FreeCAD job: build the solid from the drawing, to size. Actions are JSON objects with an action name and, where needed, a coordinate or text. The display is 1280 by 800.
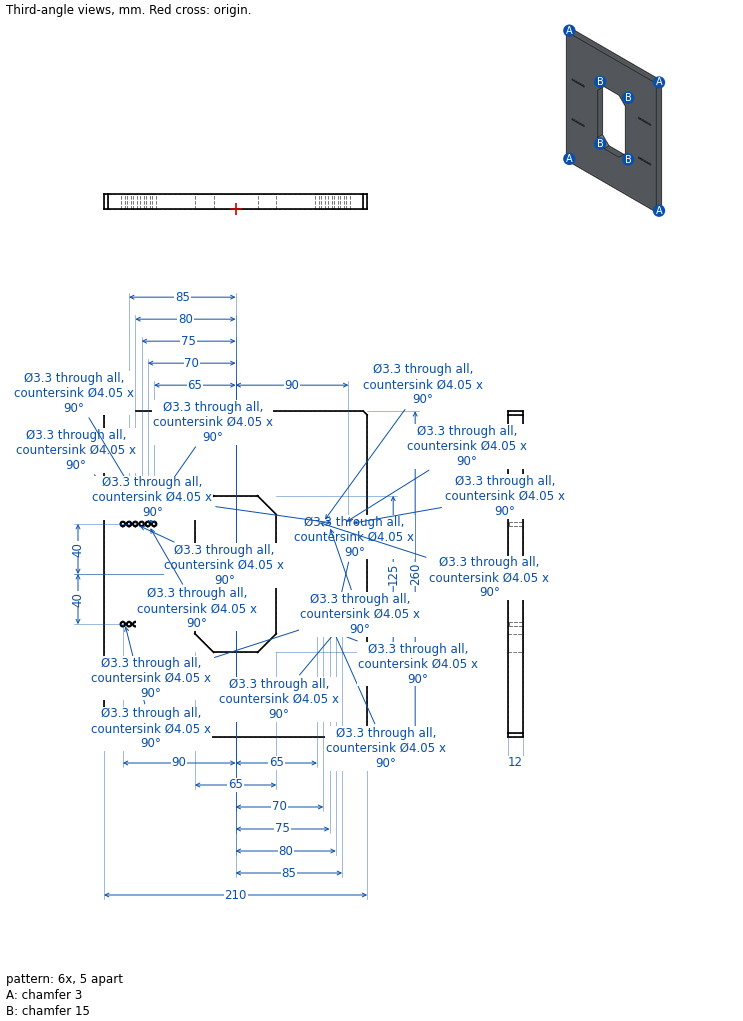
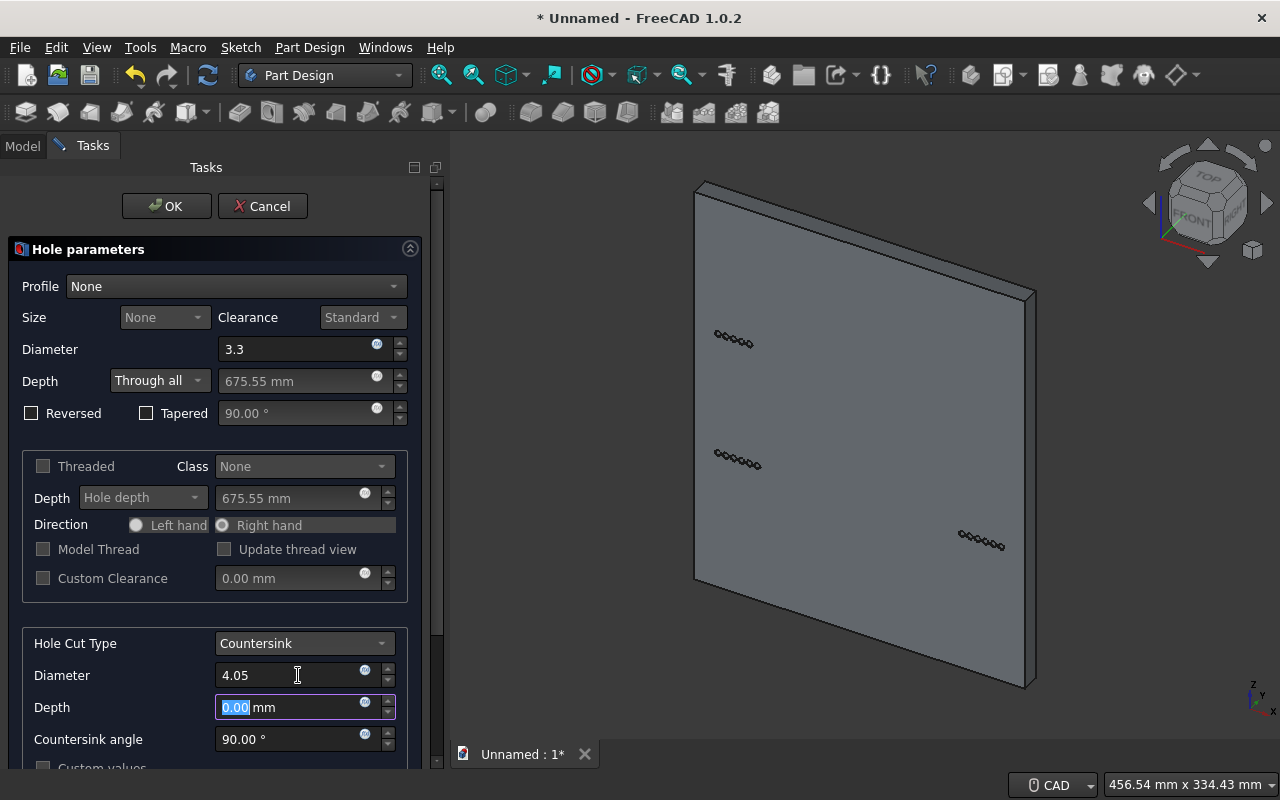
{"action": "left_click", "coordinate": [167, 206]}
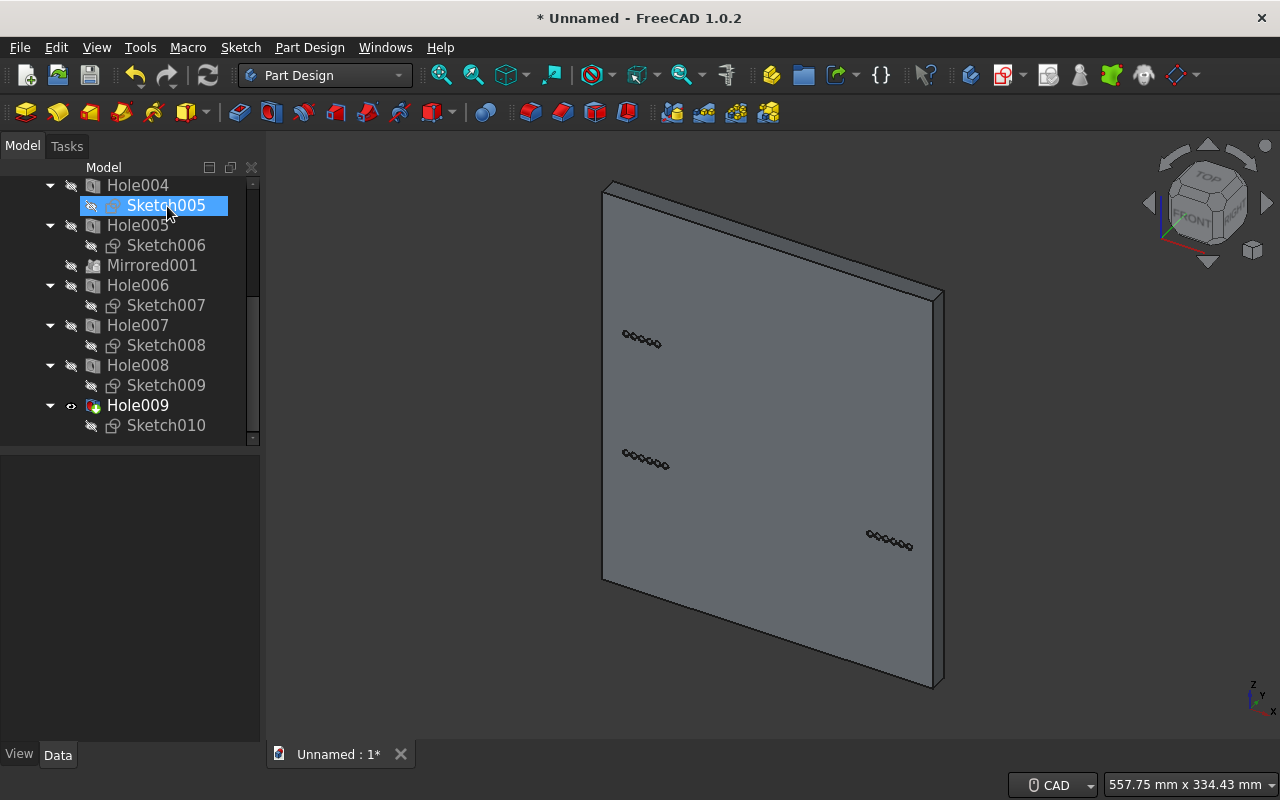
{"action": "left_click", "coordinate": [815, 400]}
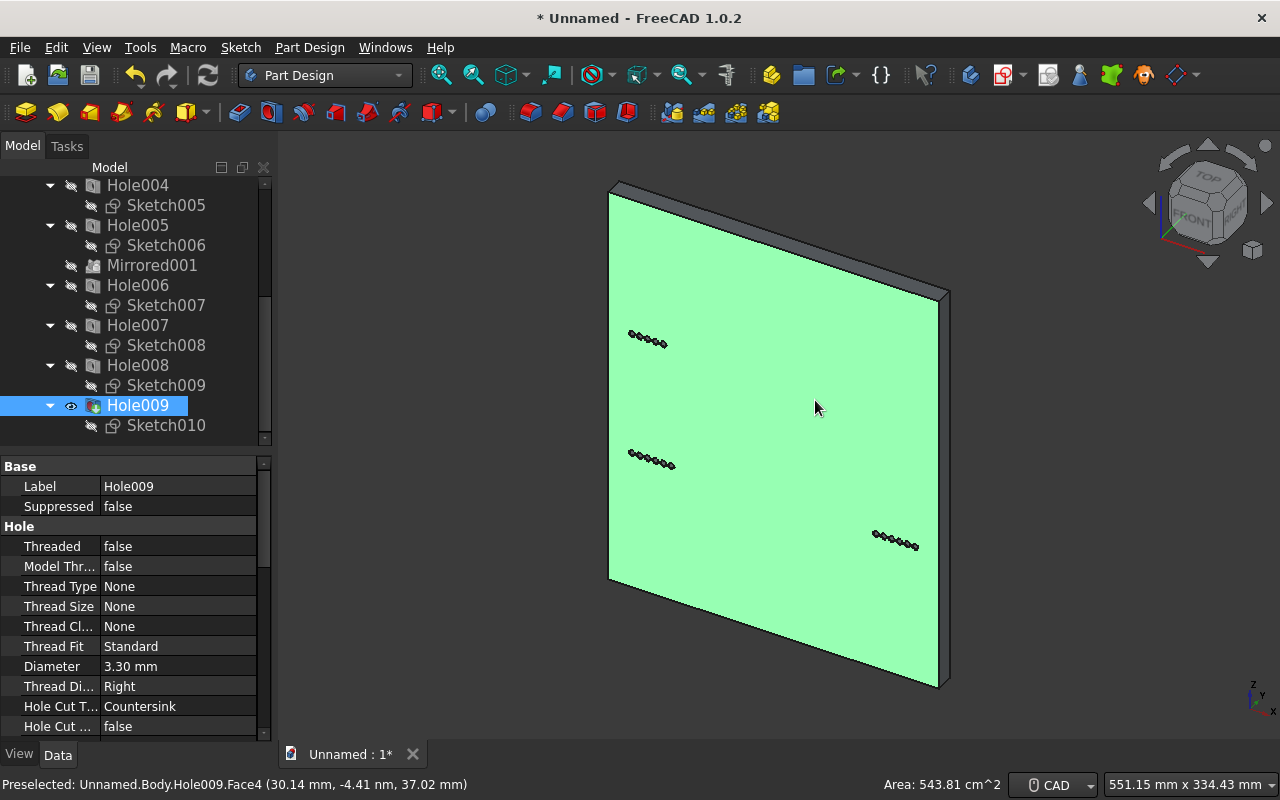
{"action": "left_click", "coordinate": [1004, 76]}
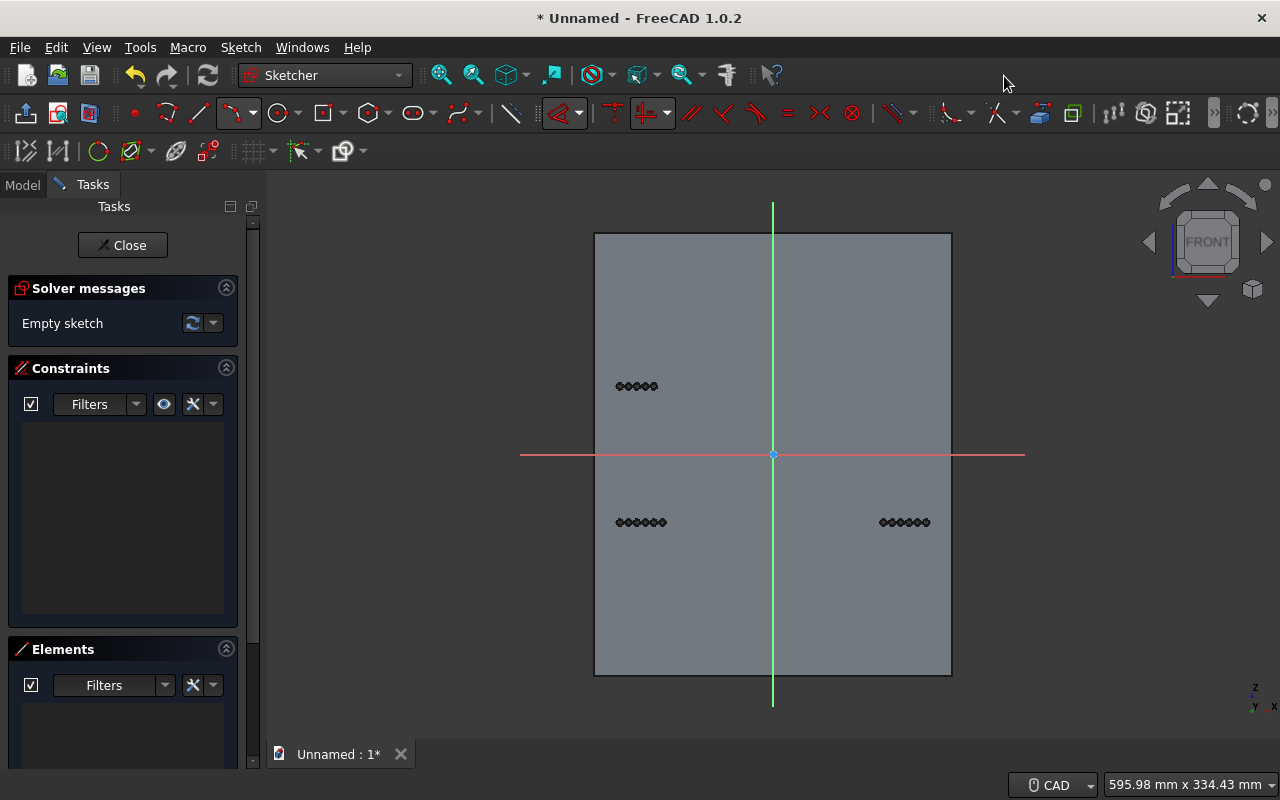
{"action": "scroll", "coordinate": [660, 383], "scroll_direction": "up", "scroll_amount": 15}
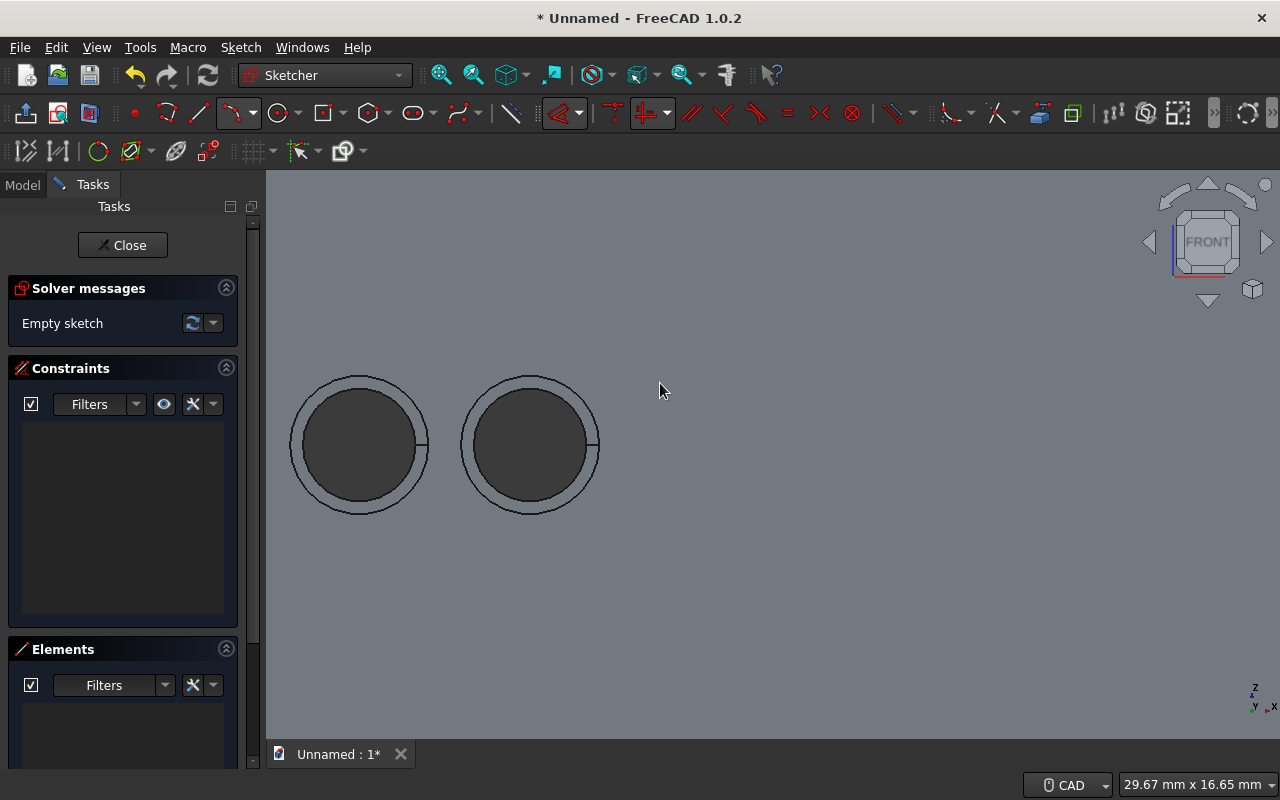
{"action": "scroll", "coordinate": [699, 441], "scroll_direction": "up", "scroll_amount": 6}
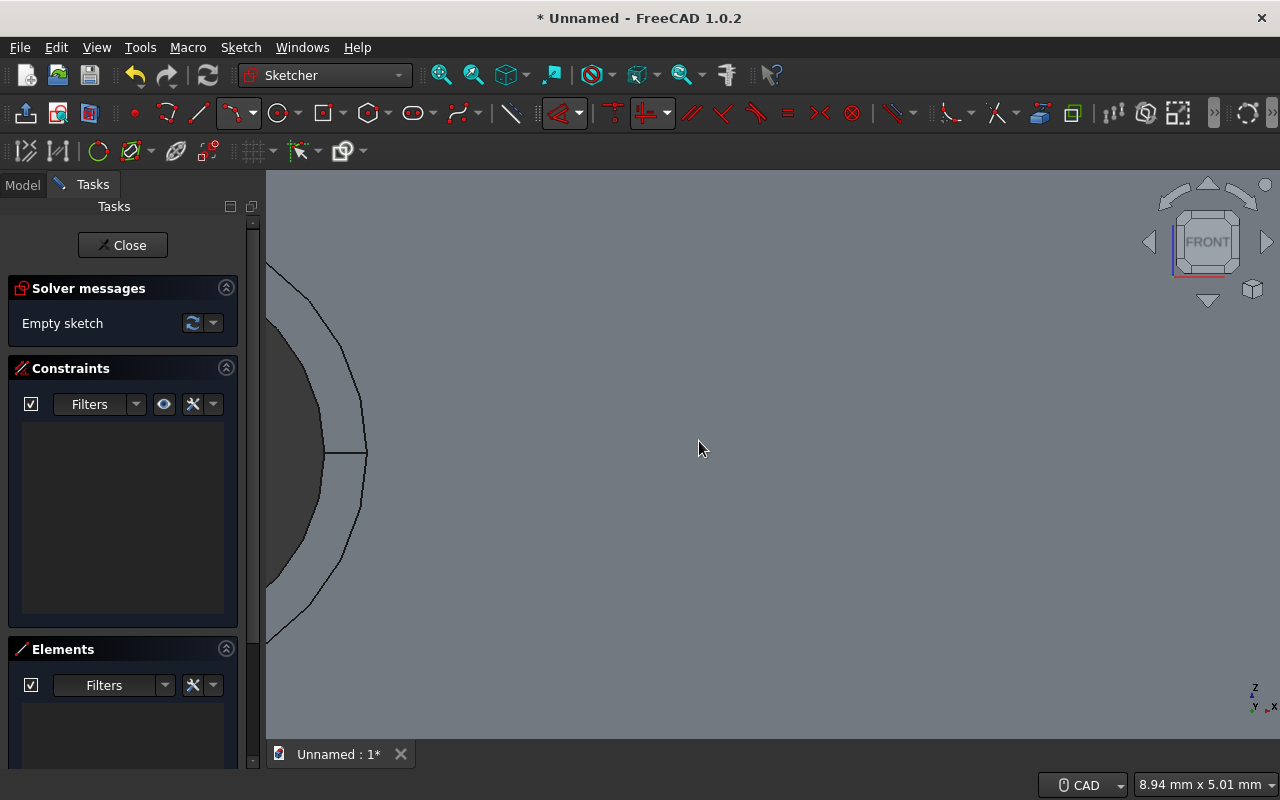
{"action": "left_click", "coordinate": [278, 114]}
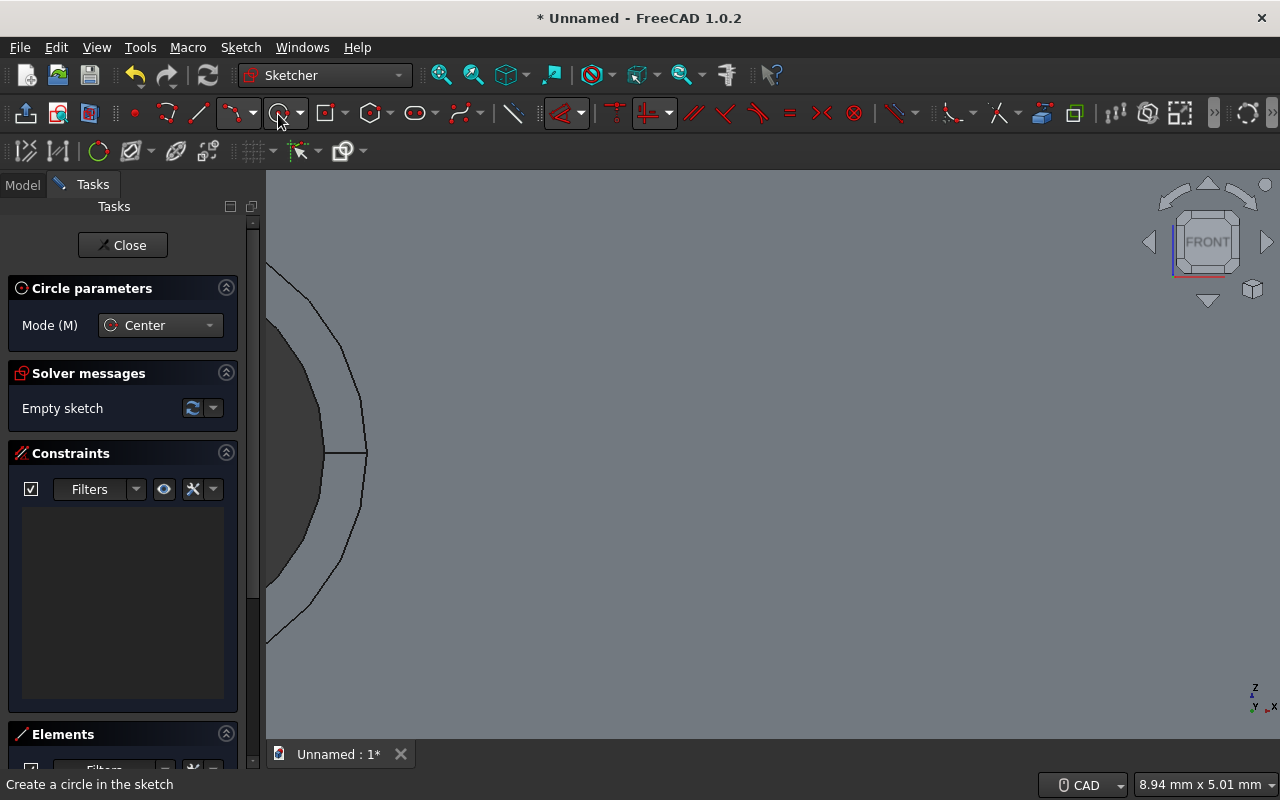
{"action": "left_click", "coordinate": [705, 453]}
{"action": "mouse_move", "coordinate": [837, 321]}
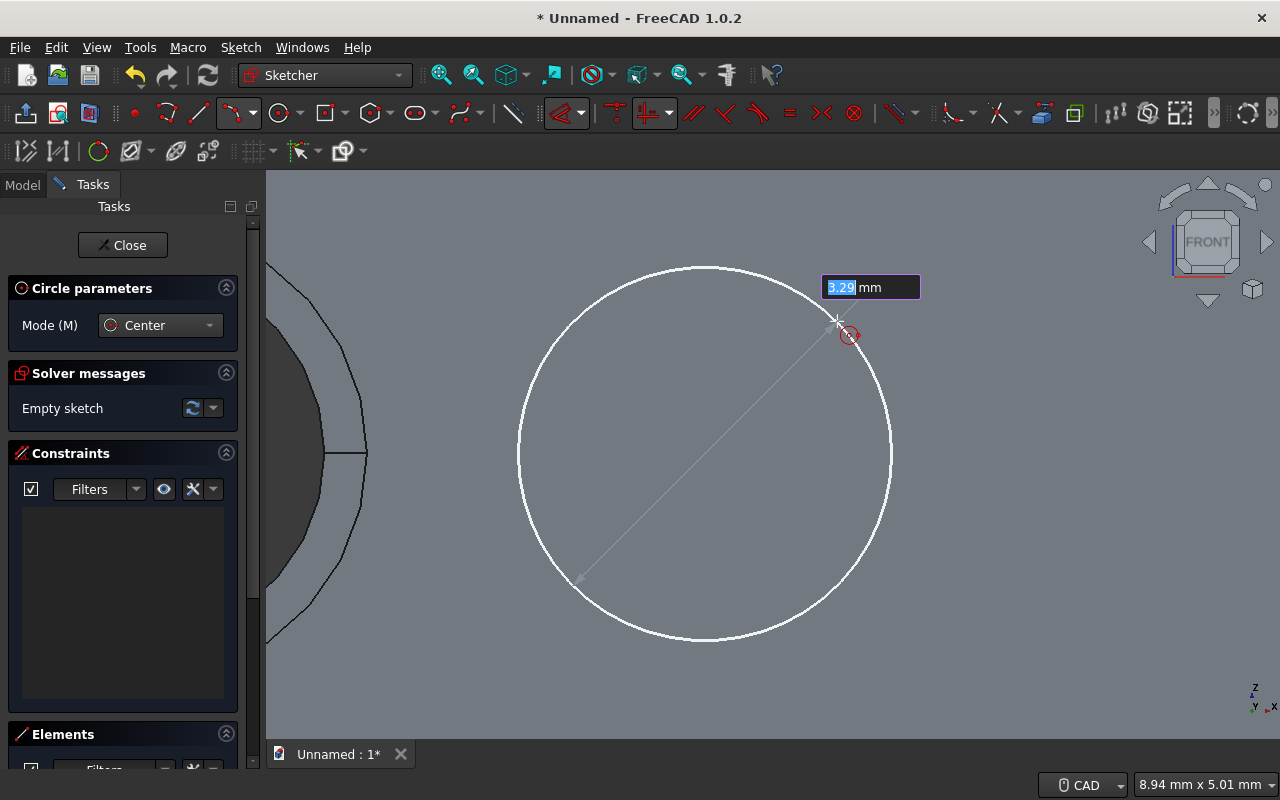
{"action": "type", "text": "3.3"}
{"action": "key", "text": "Return"}
{"action": "key", "text": "Escape"}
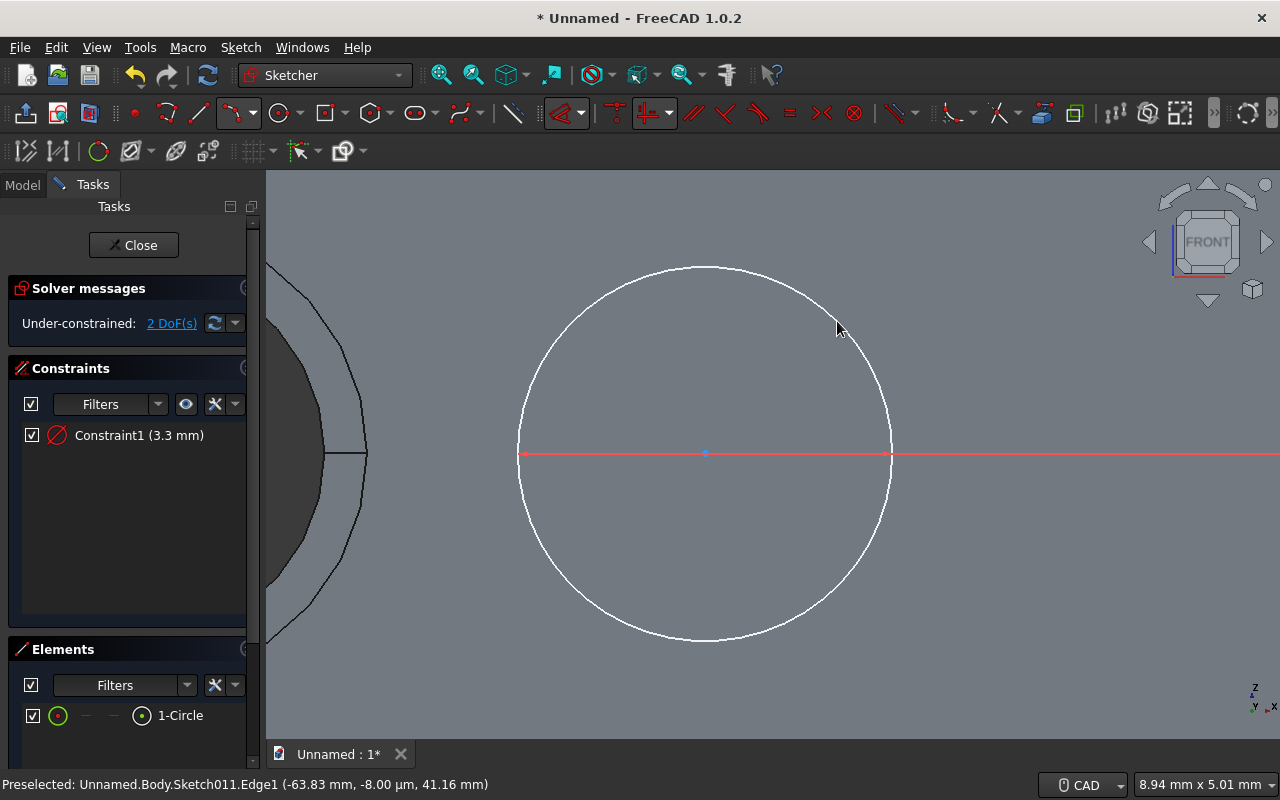
{"action": "left_click", "coordinate": [705, 454]}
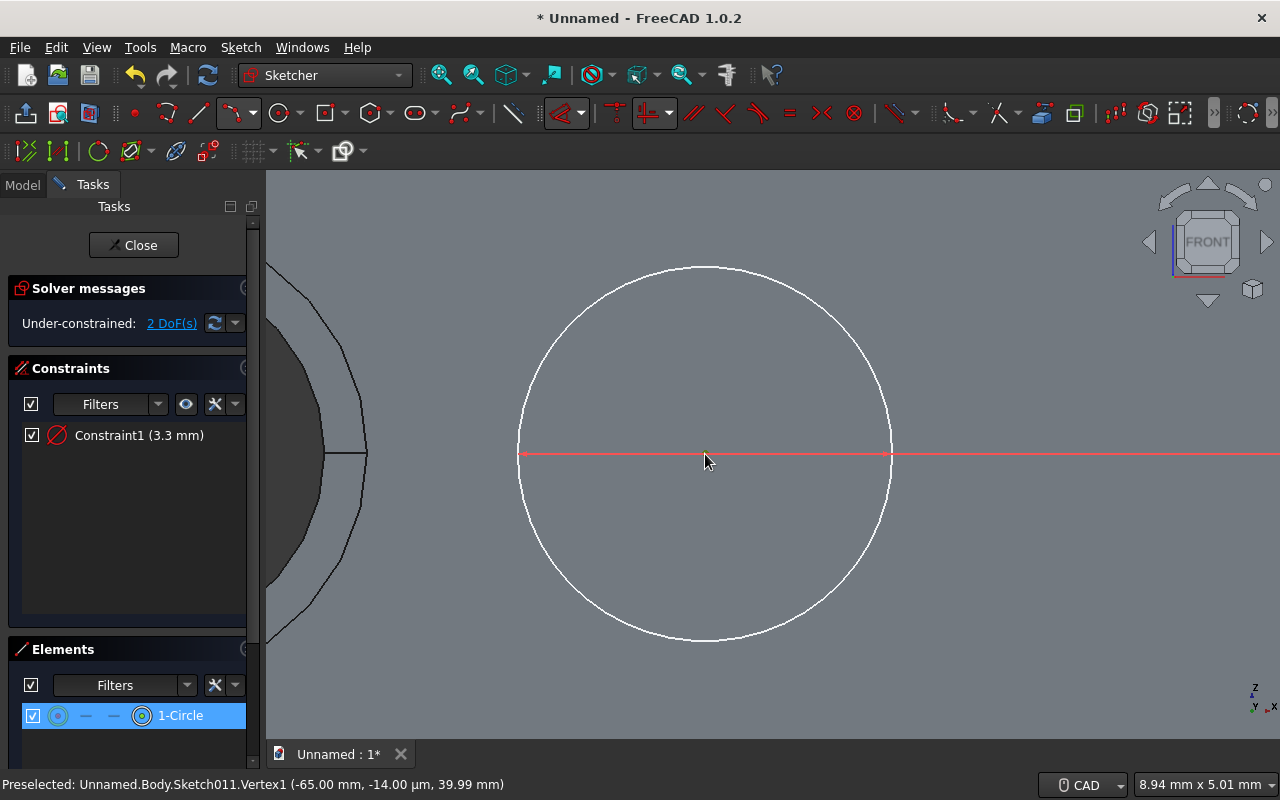
{"action": "left_click", "coordinate": [584, 114]}